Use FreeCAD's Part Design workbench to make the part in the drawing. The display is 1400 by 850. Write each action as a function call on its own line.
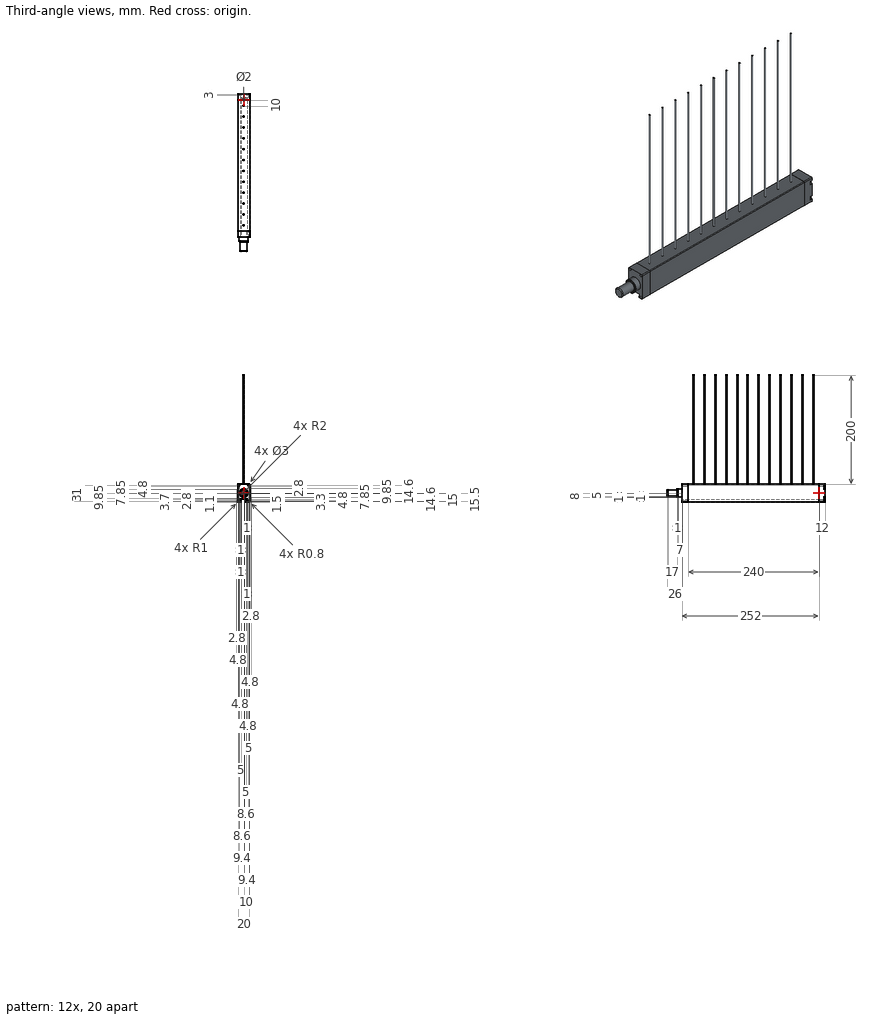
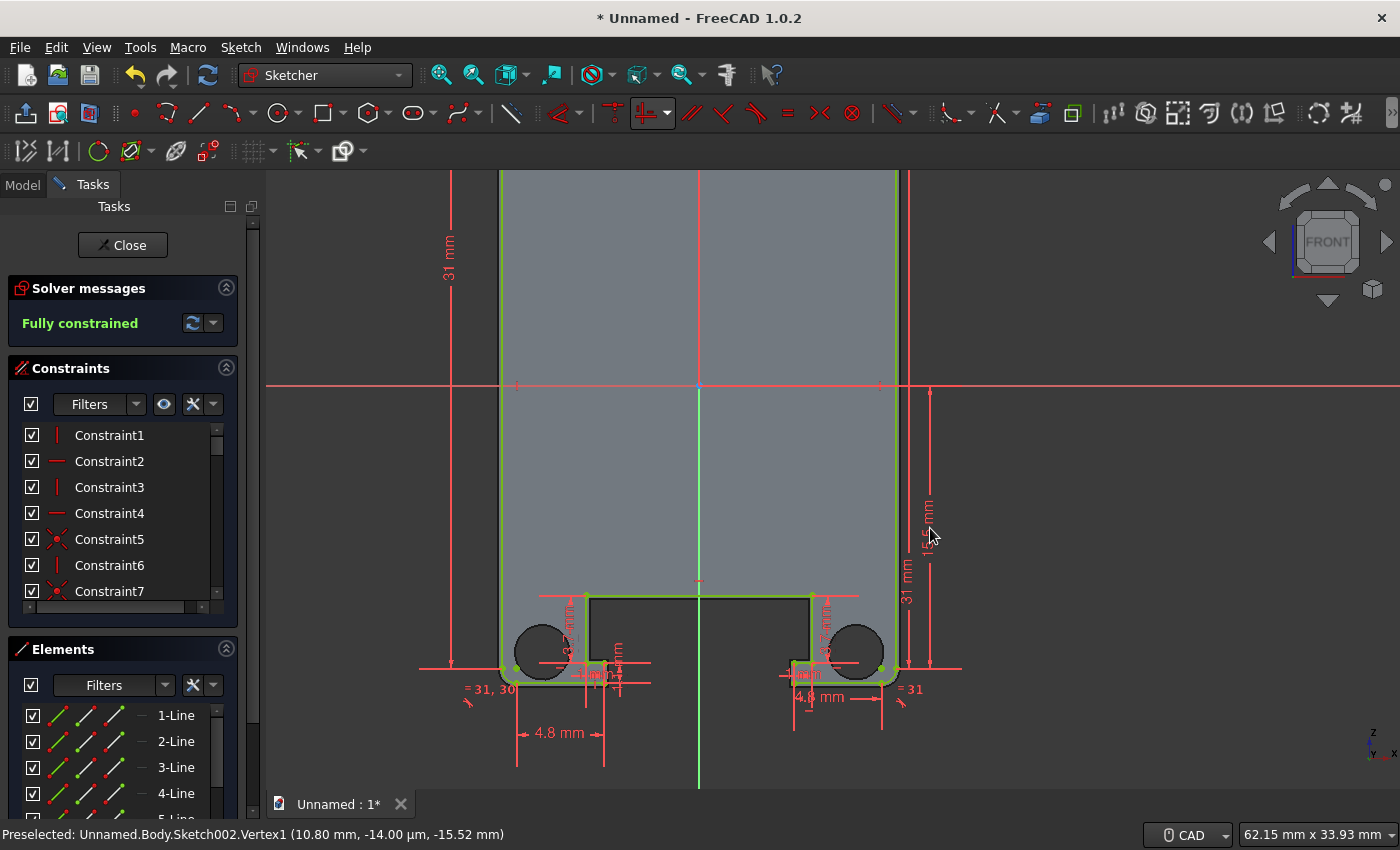
click(123, 245)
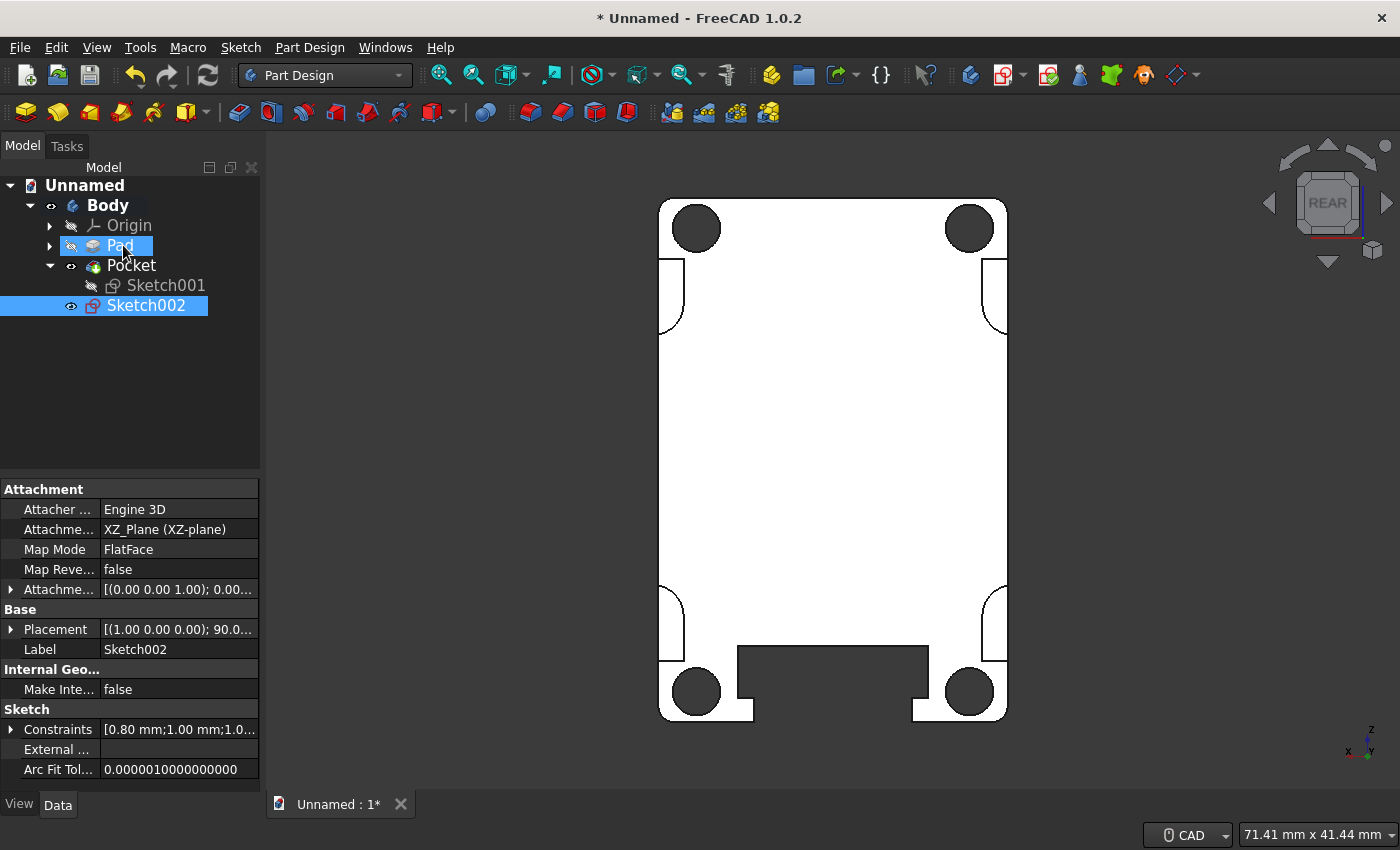
click(26, 112)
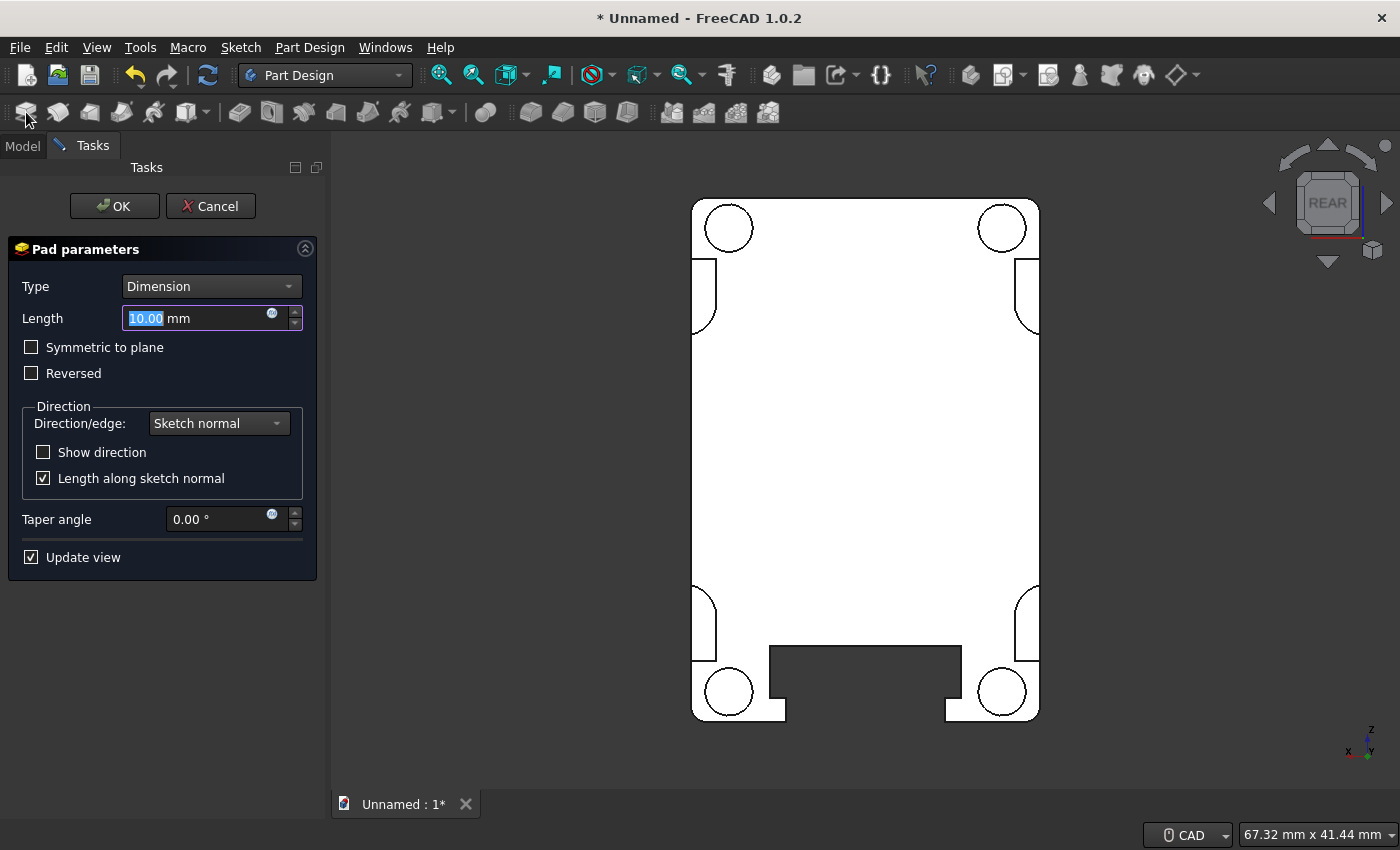
text(240)
key(Tab)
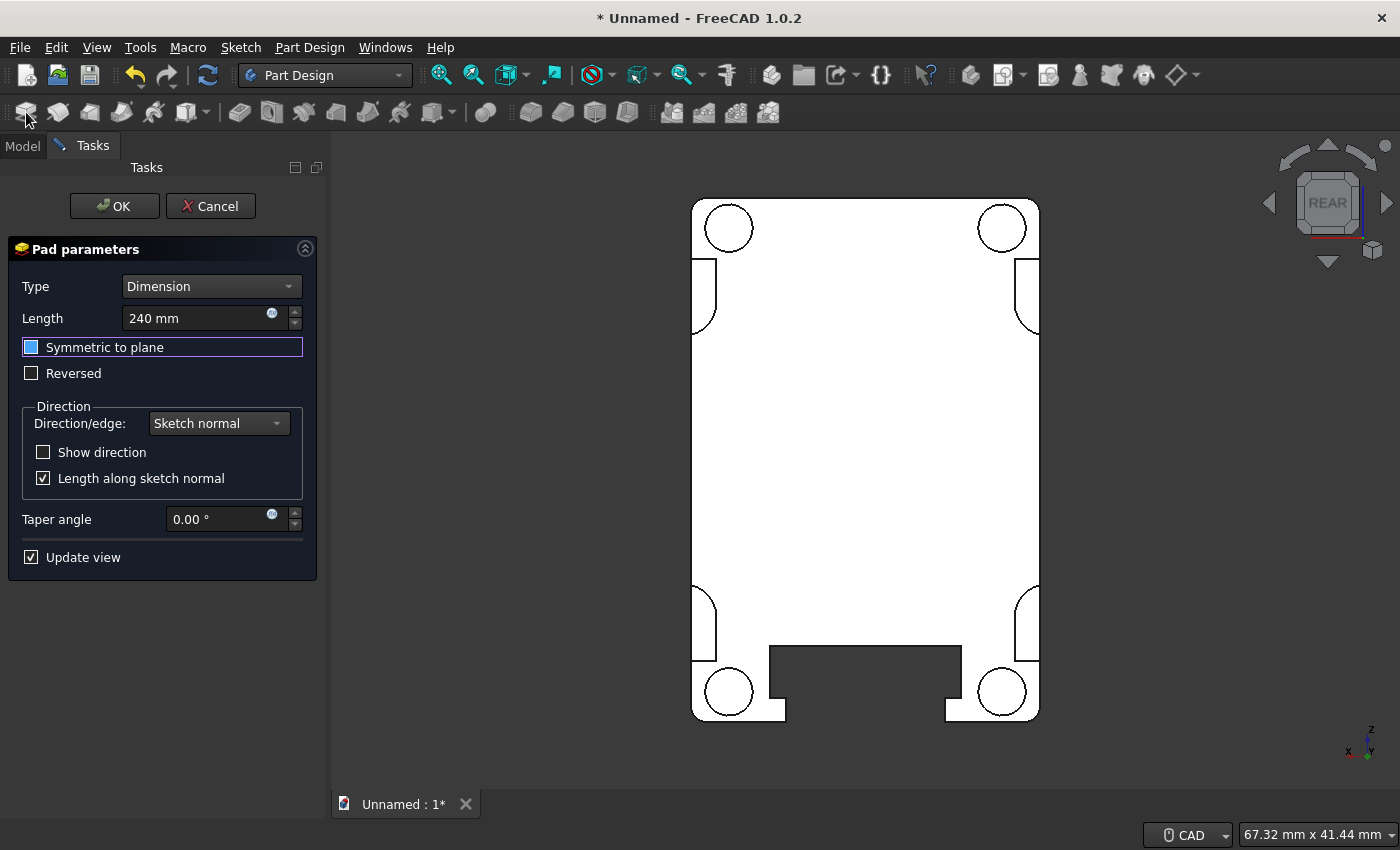
click(115, 206)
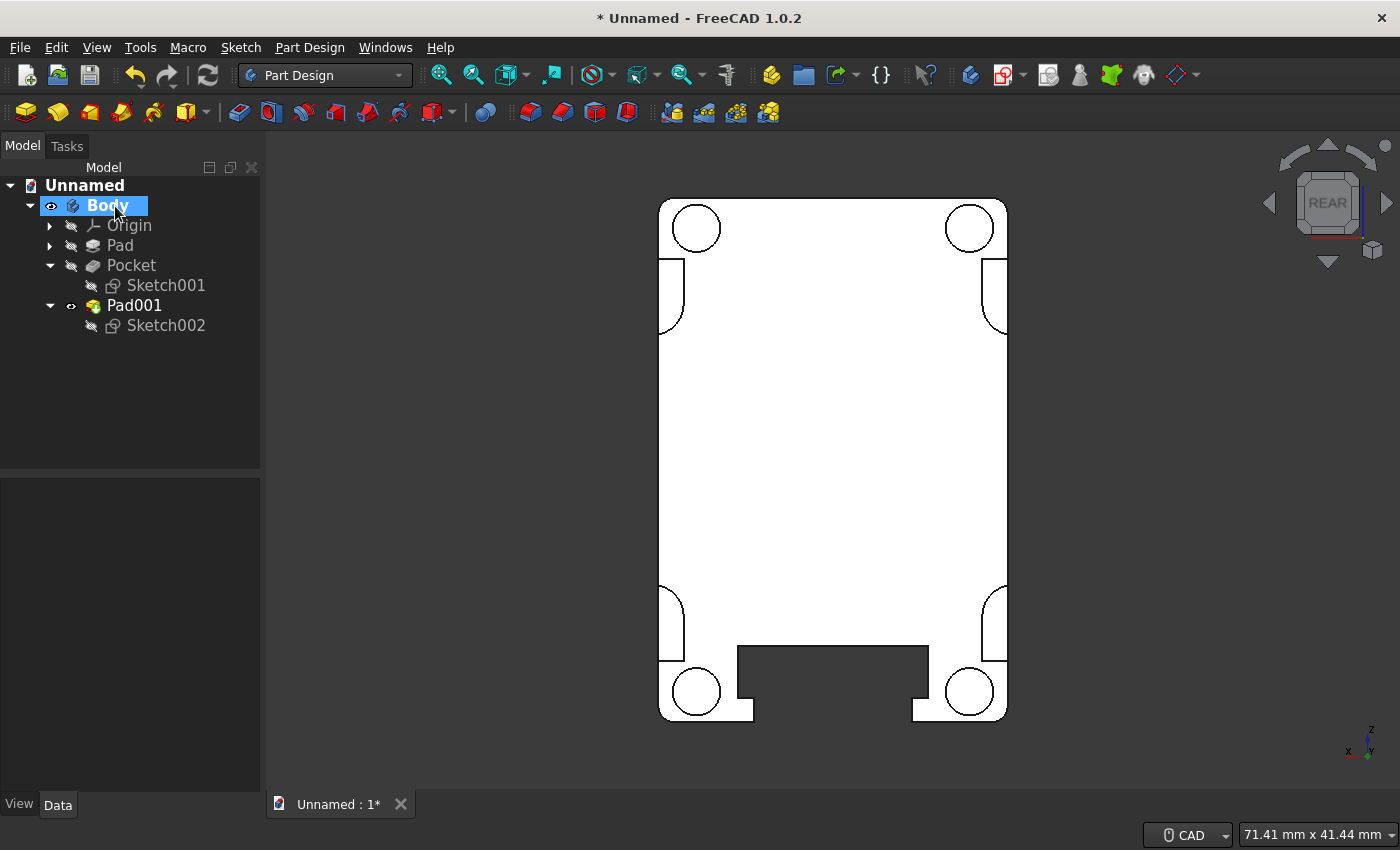
click(50, 226)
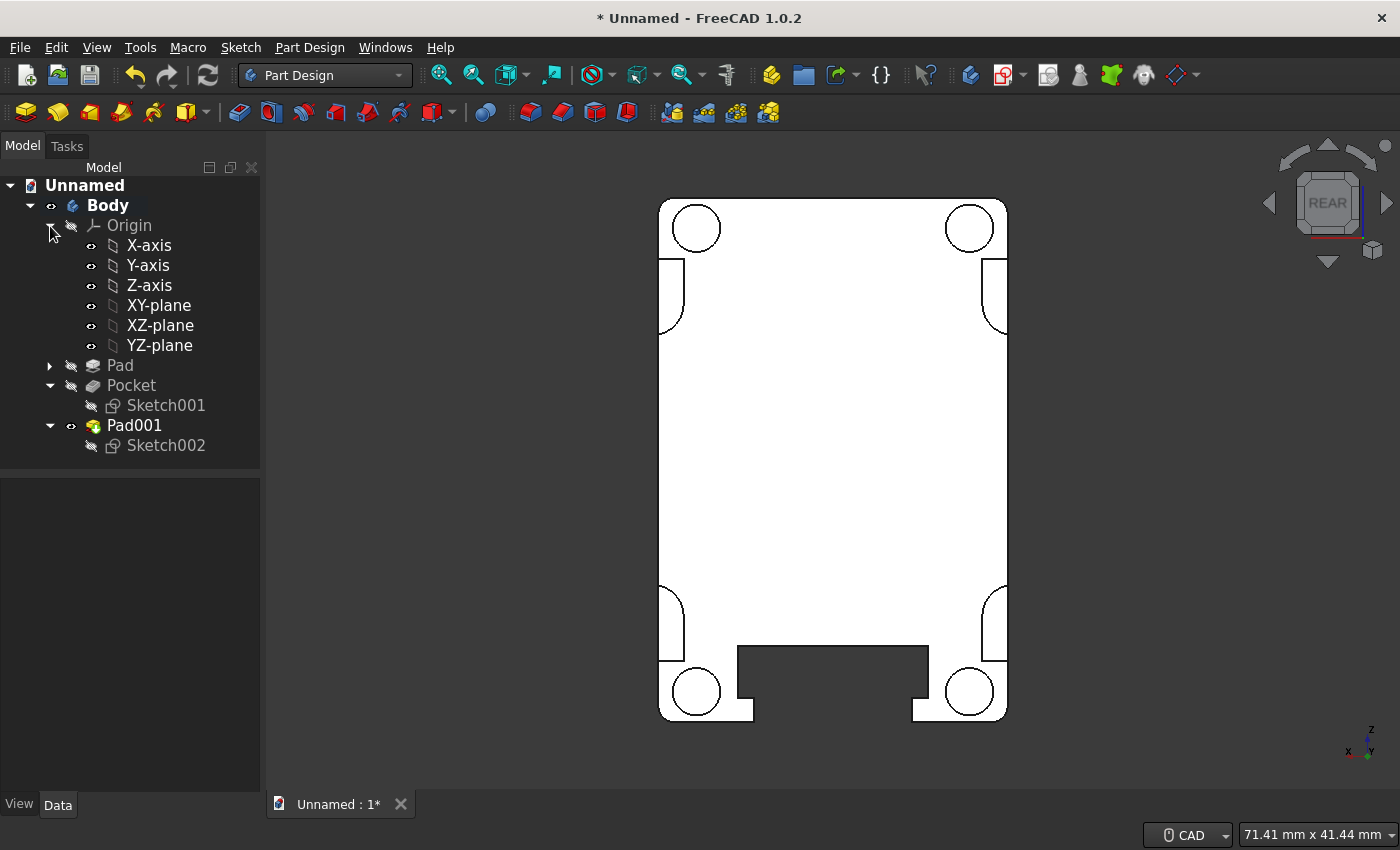
click(136, 326)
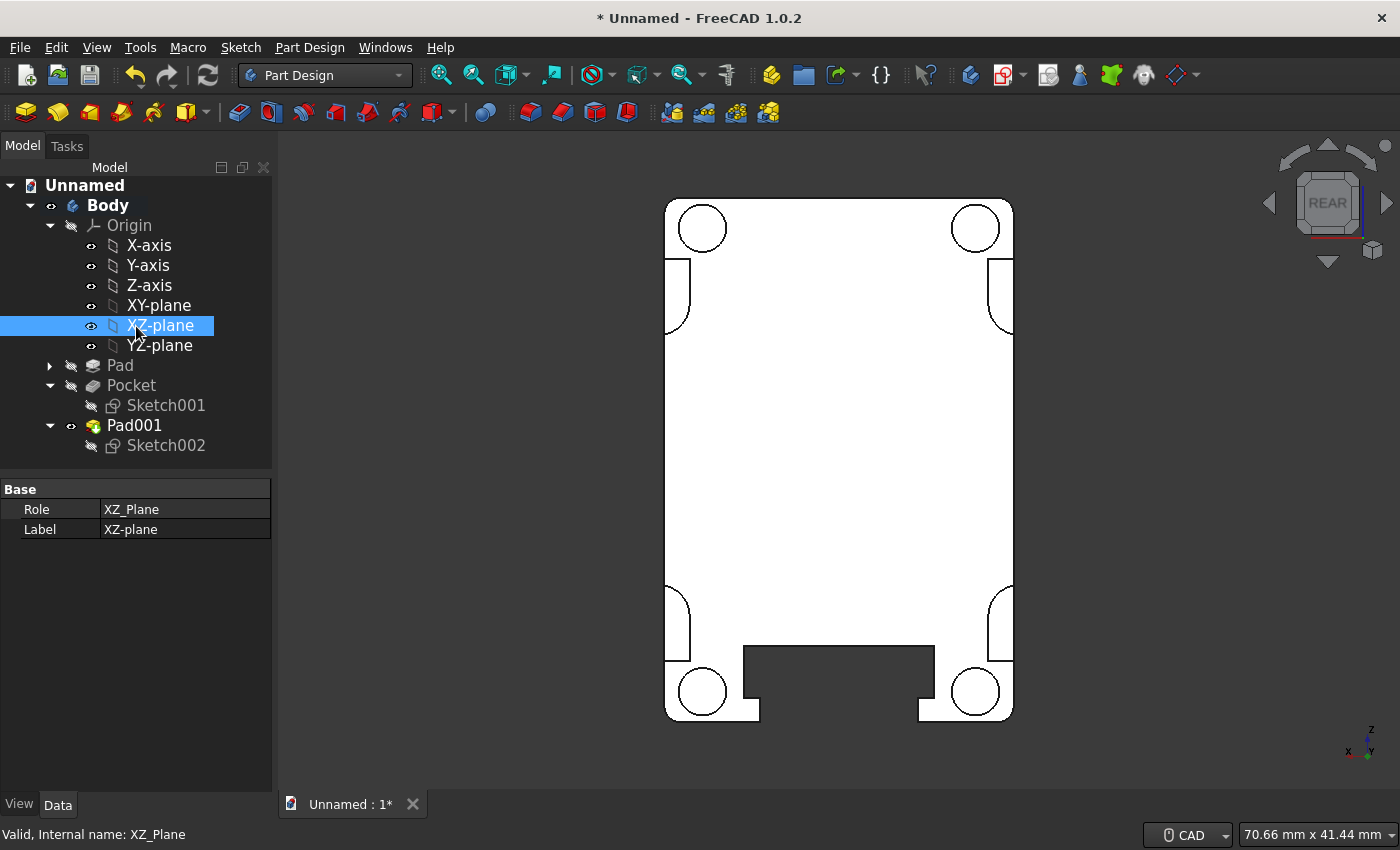
click(1176, 76)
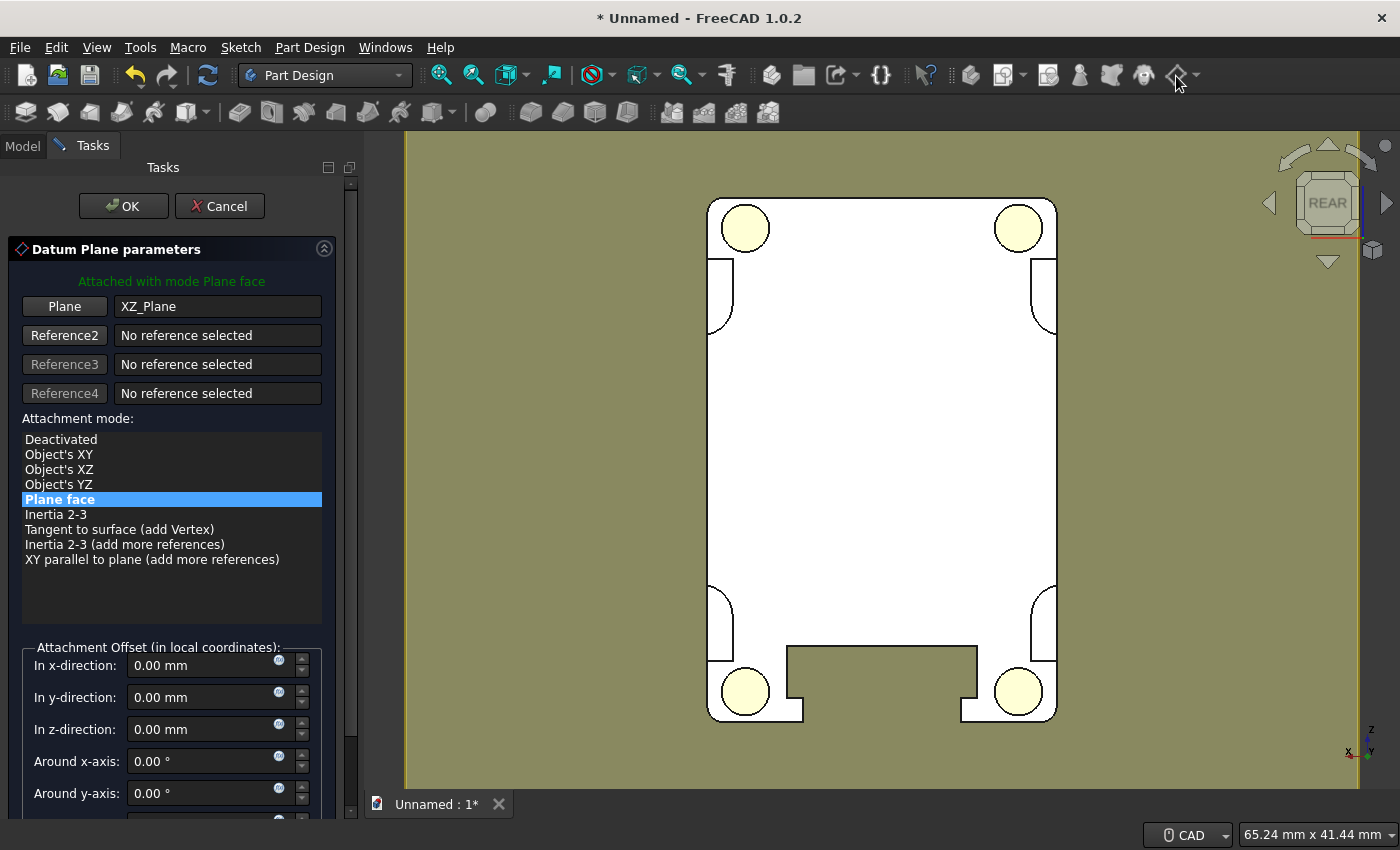
triple_click(210, 729)